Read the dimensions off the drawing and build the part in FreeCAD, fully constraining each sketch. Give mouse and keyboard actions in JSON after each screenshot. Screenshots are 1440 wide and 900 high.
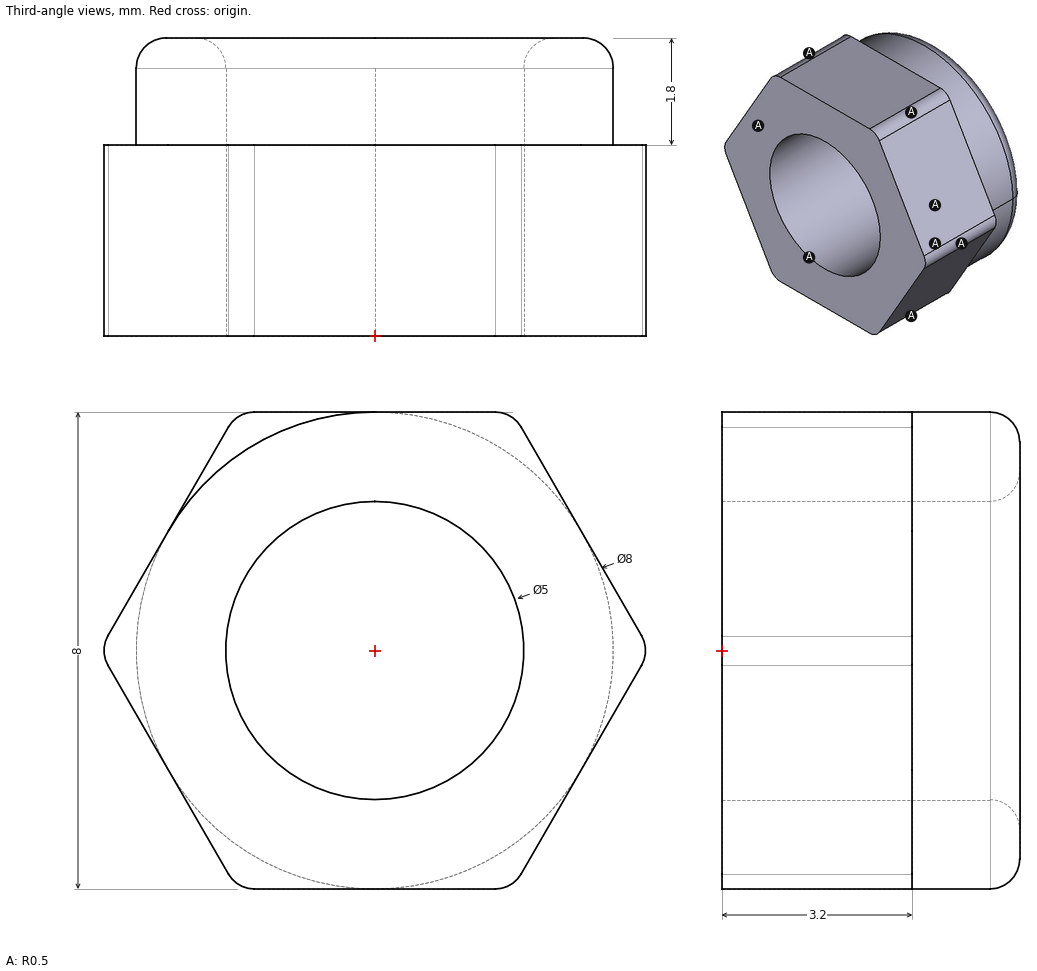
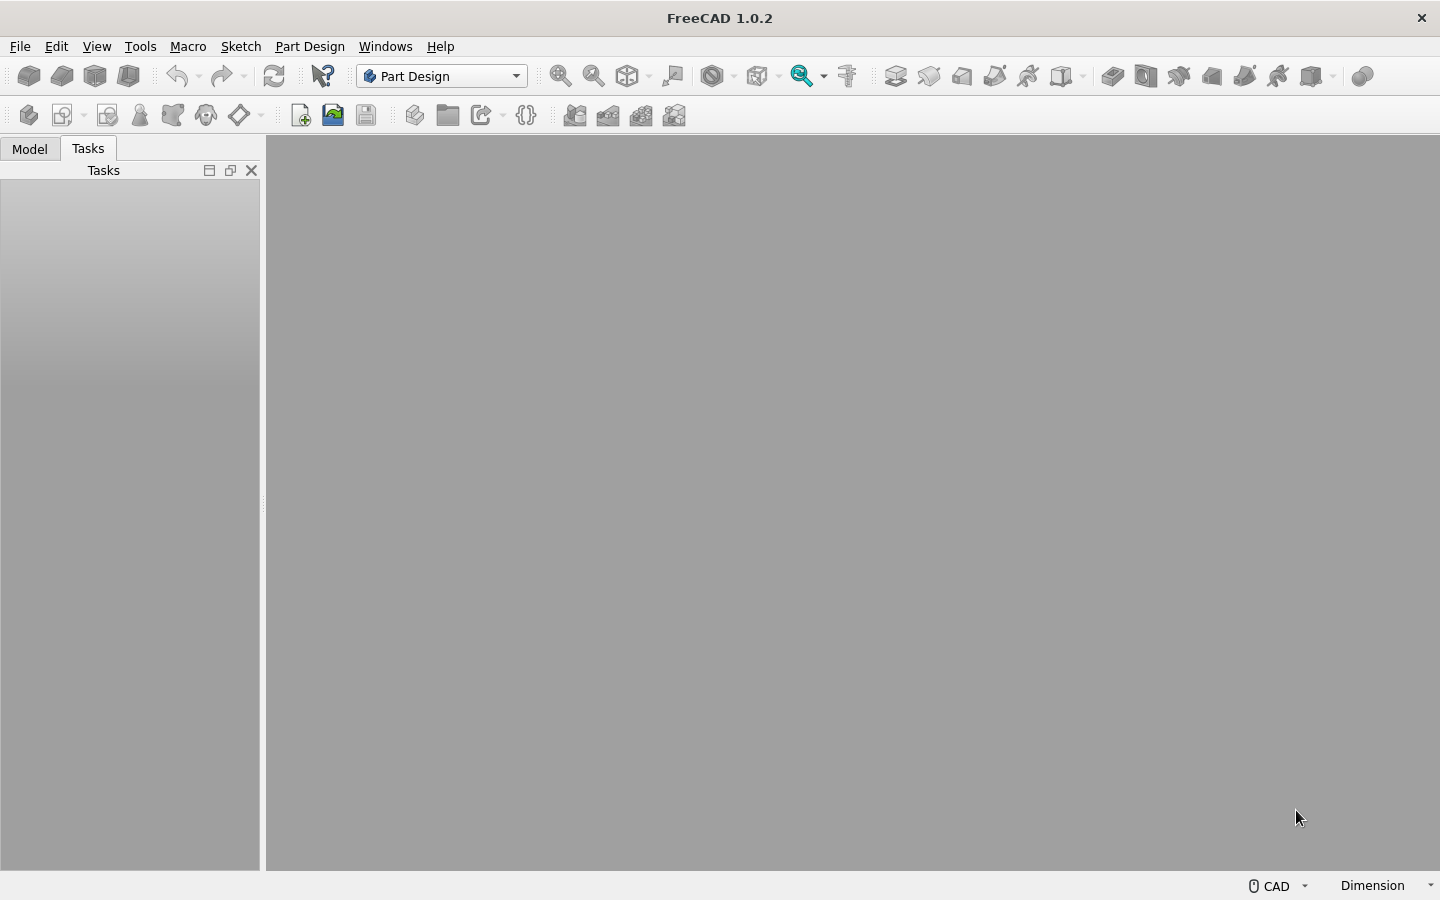
{"action": "left_click", "coordinate": [300, 116]}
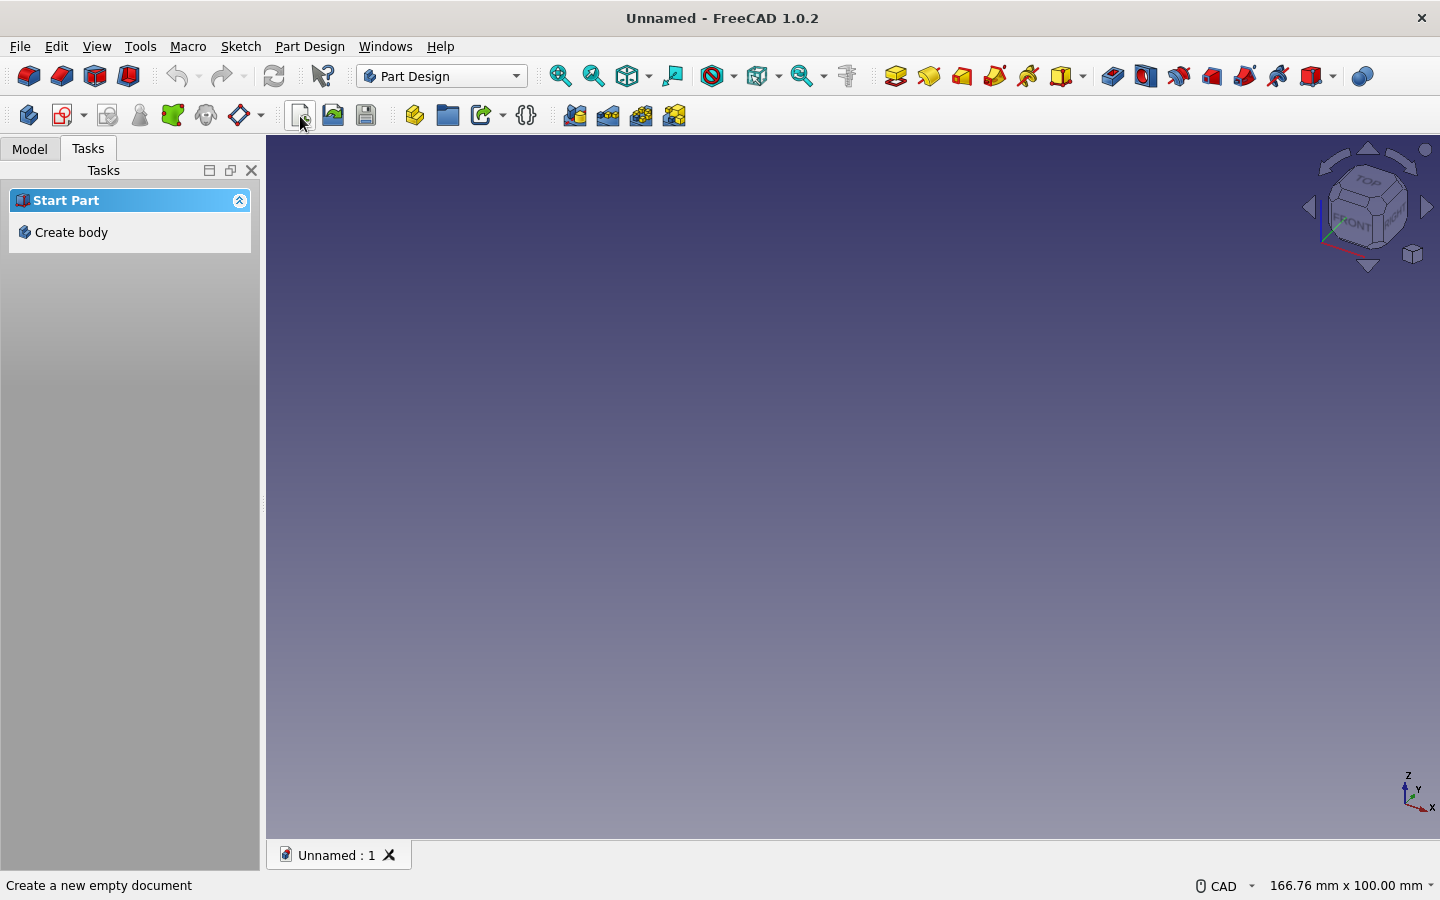
{"action": "left_click", "coordinate": [62, 116]}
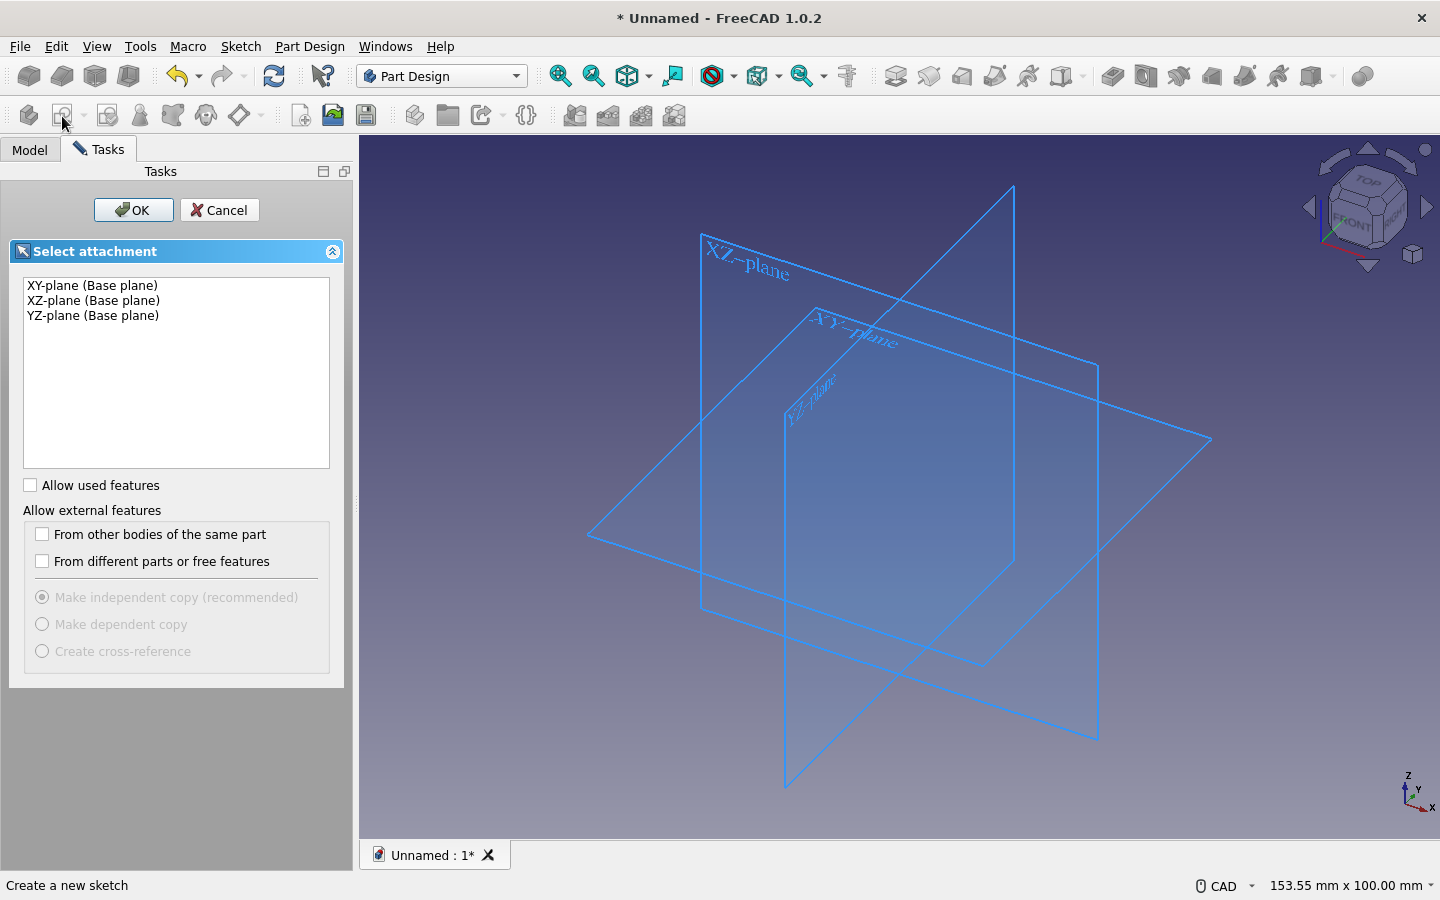
{"action": "left_click", "coordinate": [84, 300]}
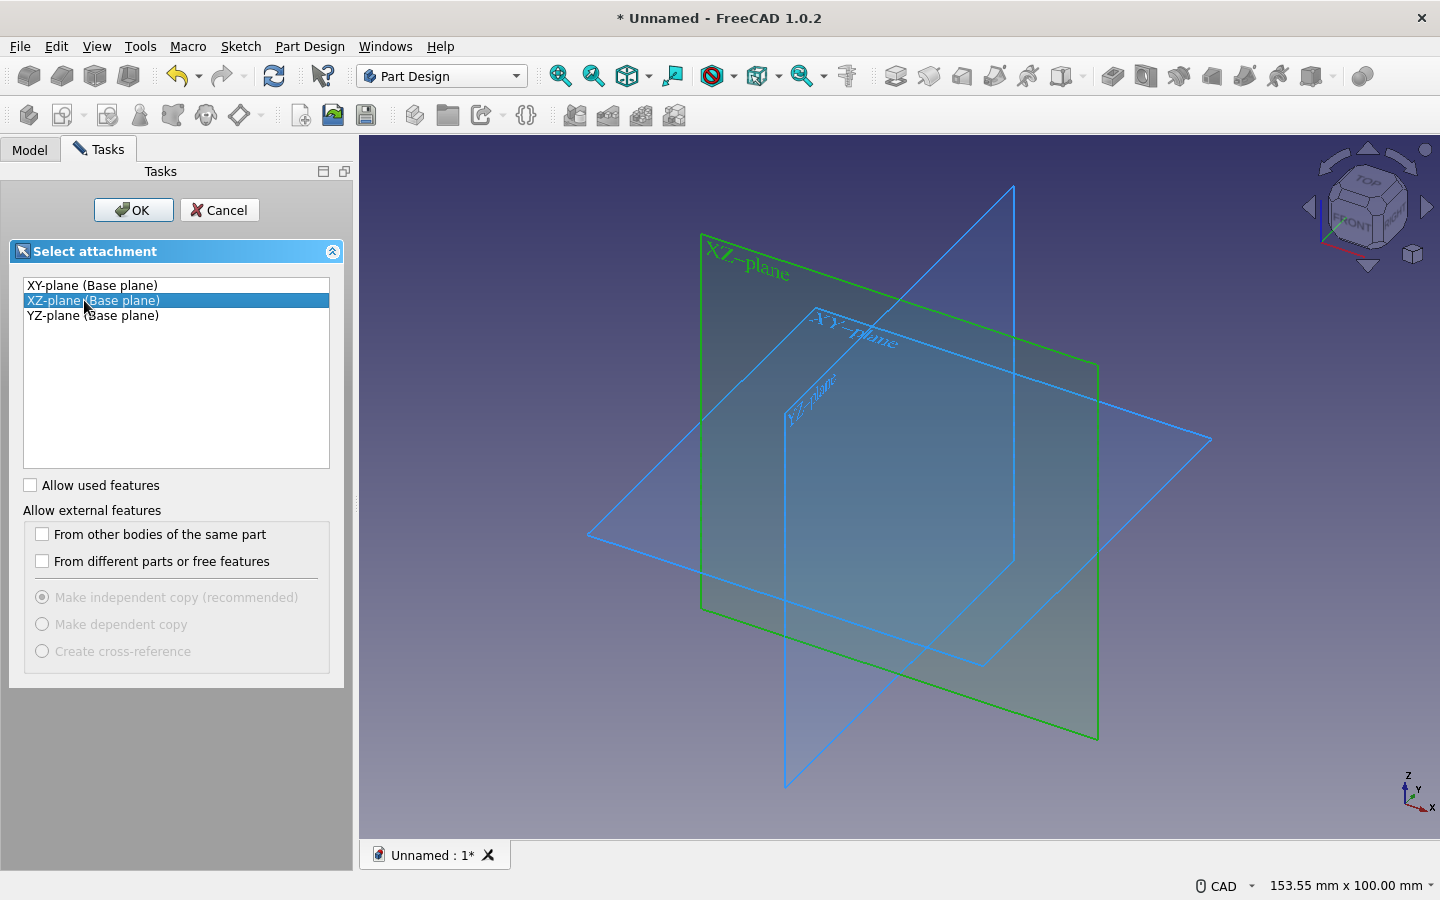
{"action": "left_click", "coordinate": [134, 210]}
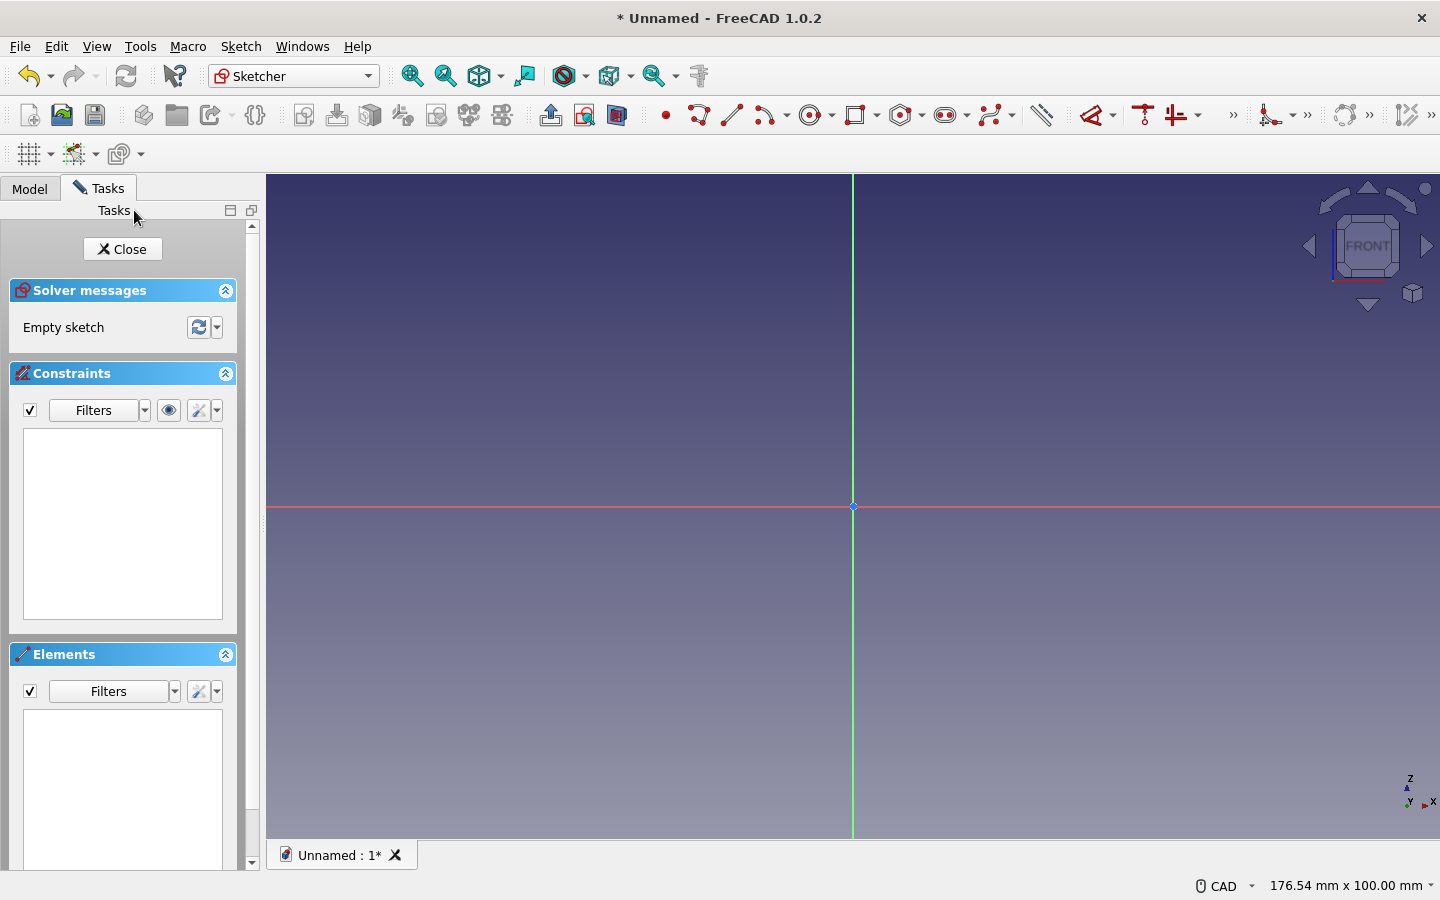
{"action": "scroll", "coordinate": [864, 506], "scroll_direction": "up", "scroll_amount": 10}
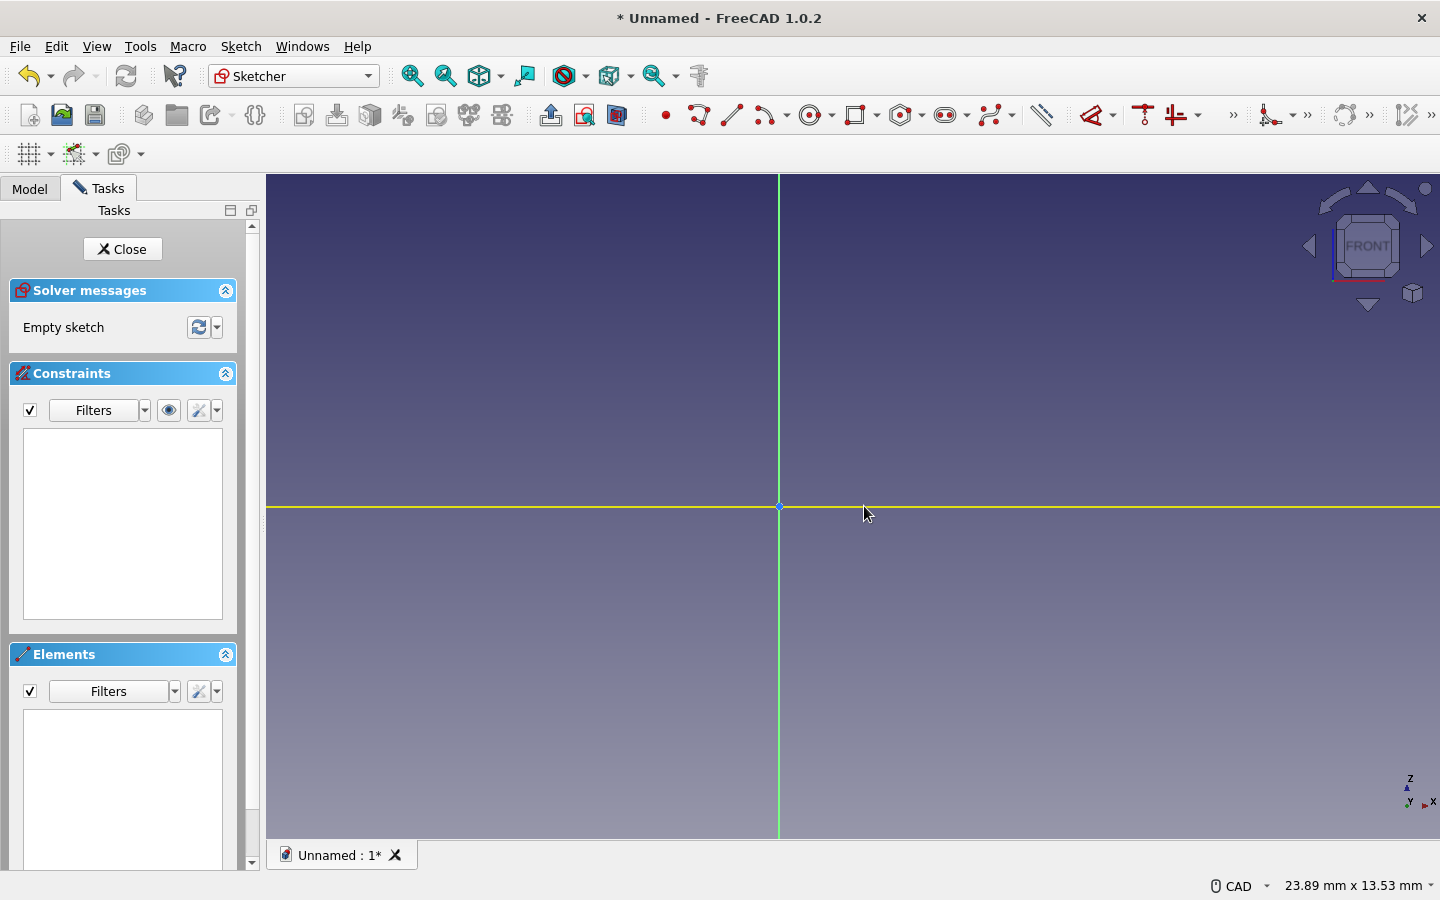
{"action": "left_click", "coordinate": [900, 116]}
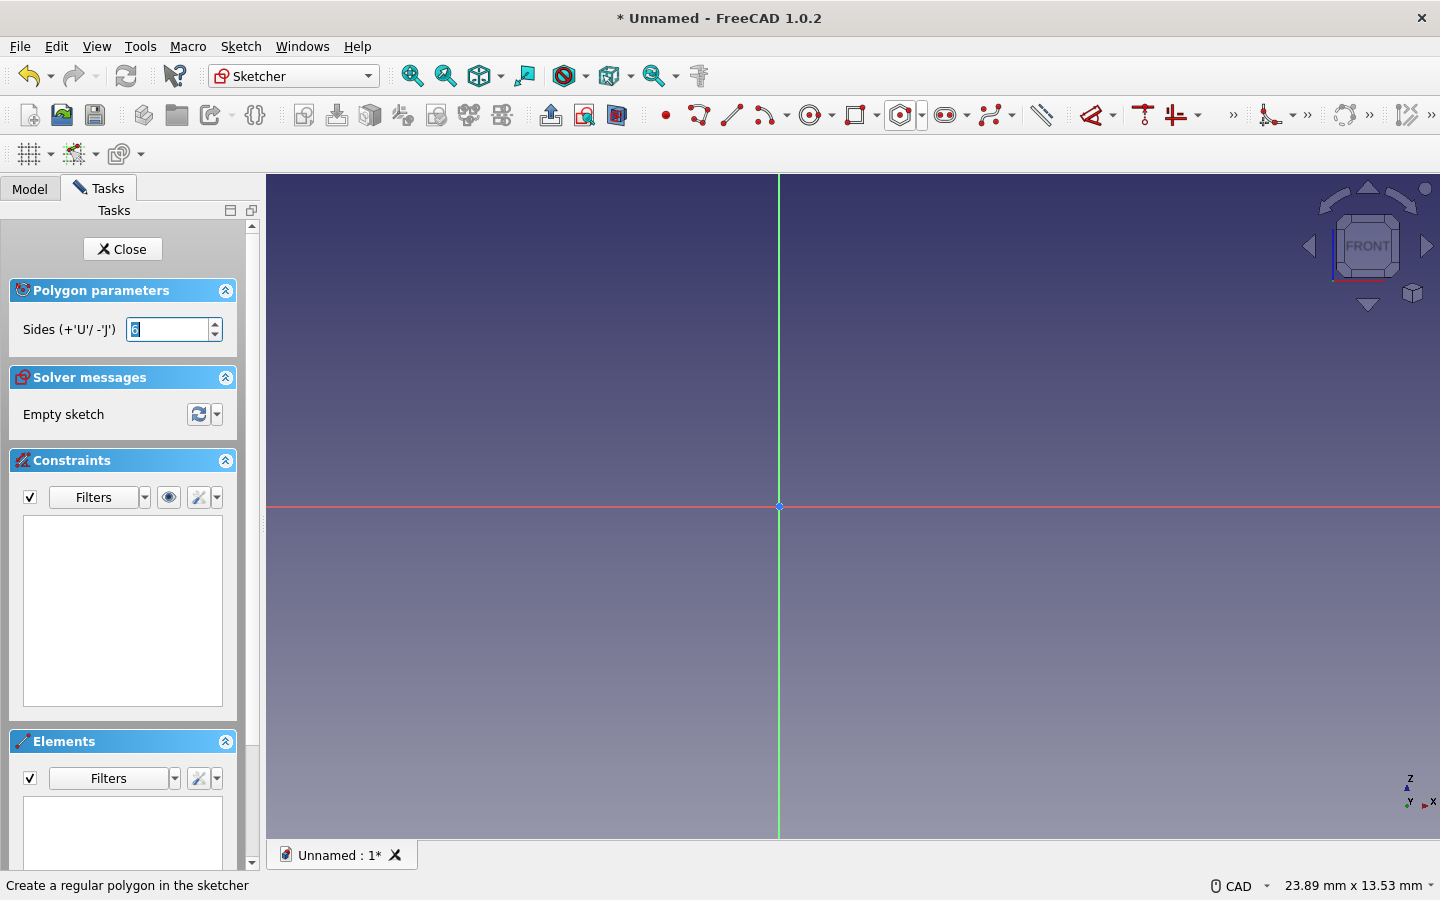
{"action": "left_click", "coordinate": [779, 506]}